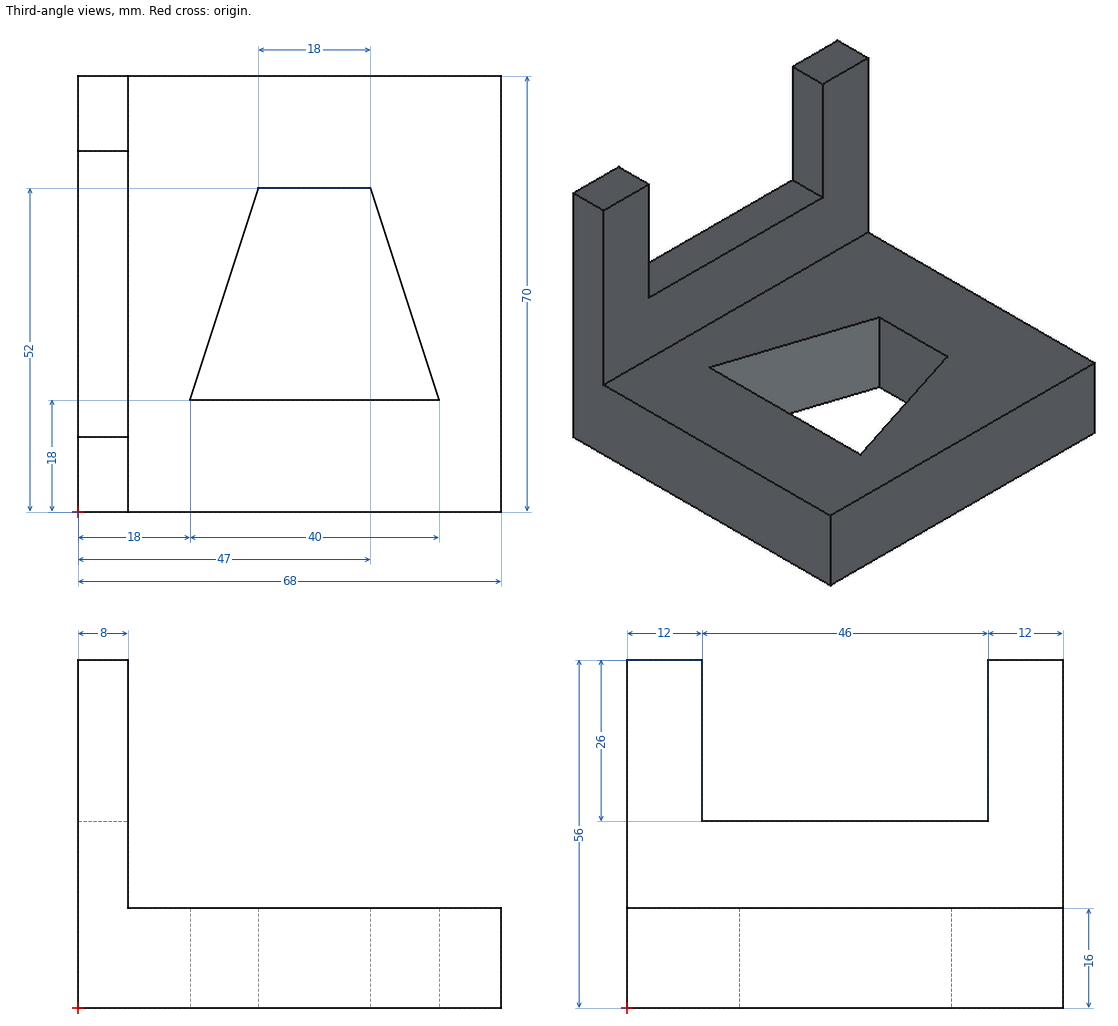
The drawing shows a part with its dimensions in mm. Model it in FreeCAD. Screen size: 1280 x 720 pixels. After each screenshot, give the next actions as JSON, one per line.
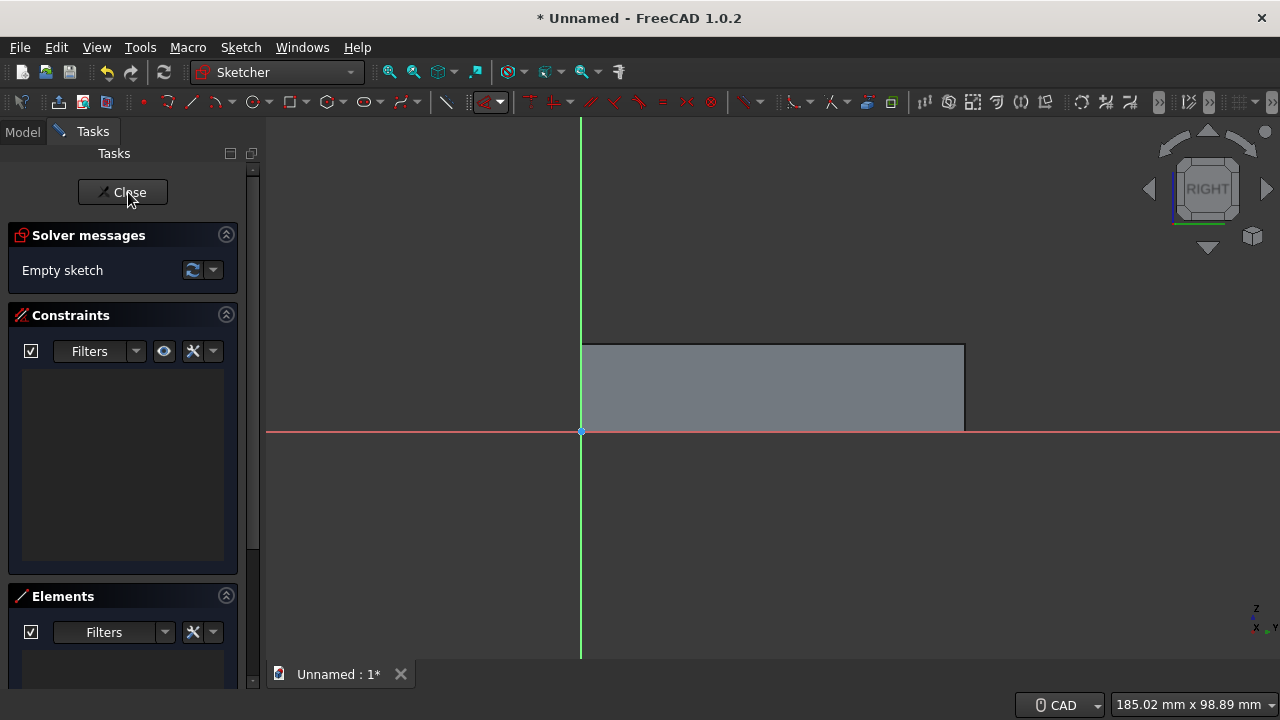
{"action": "scroll", "coordinate": [395, 631], "scroll_direction": "down", "scroll_amount": 1}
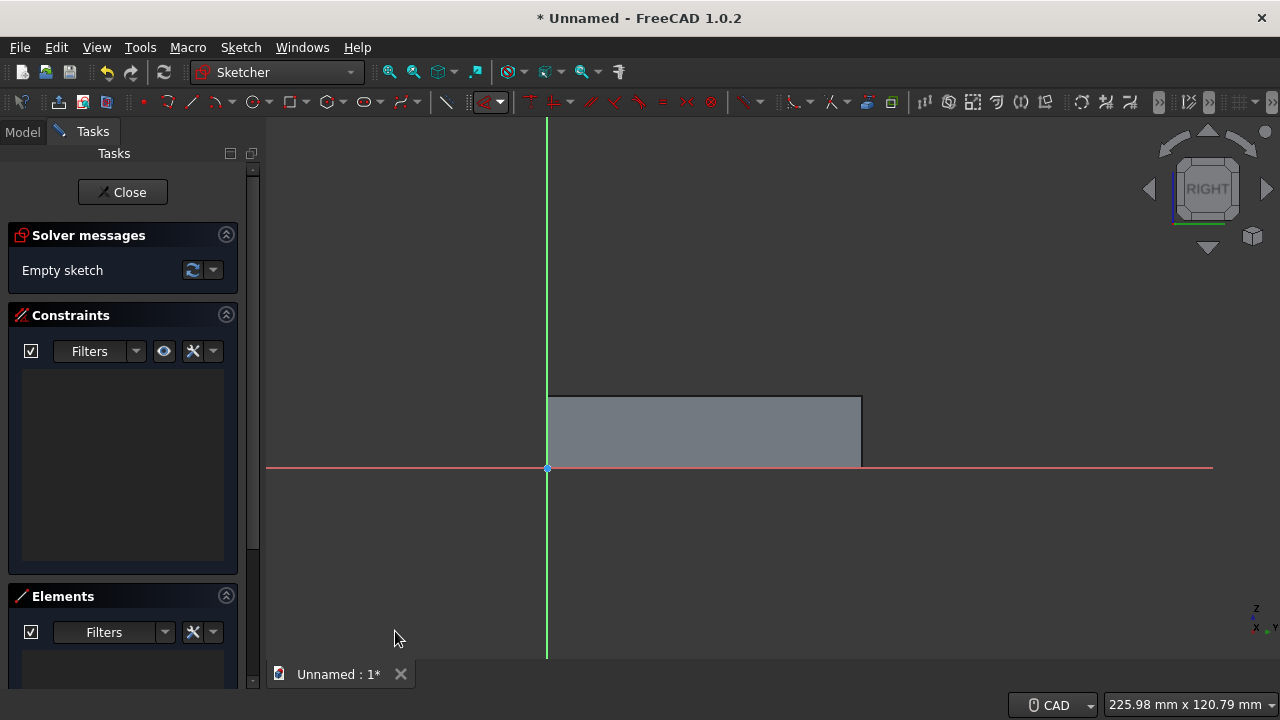
{"action": "scroll", "coordinate": [705, 250], "scroll_direction": "up", "scroll_amount": 2}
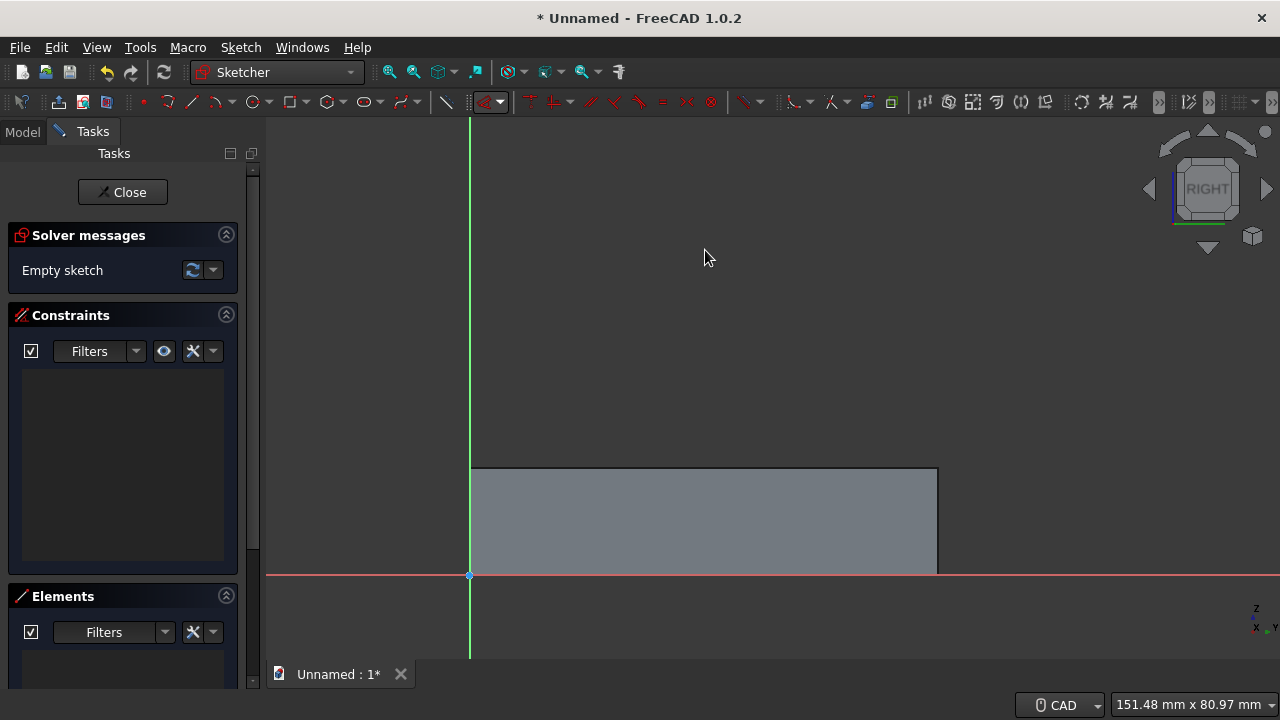
{"action": "left_click", "coordinate": [168, 102]}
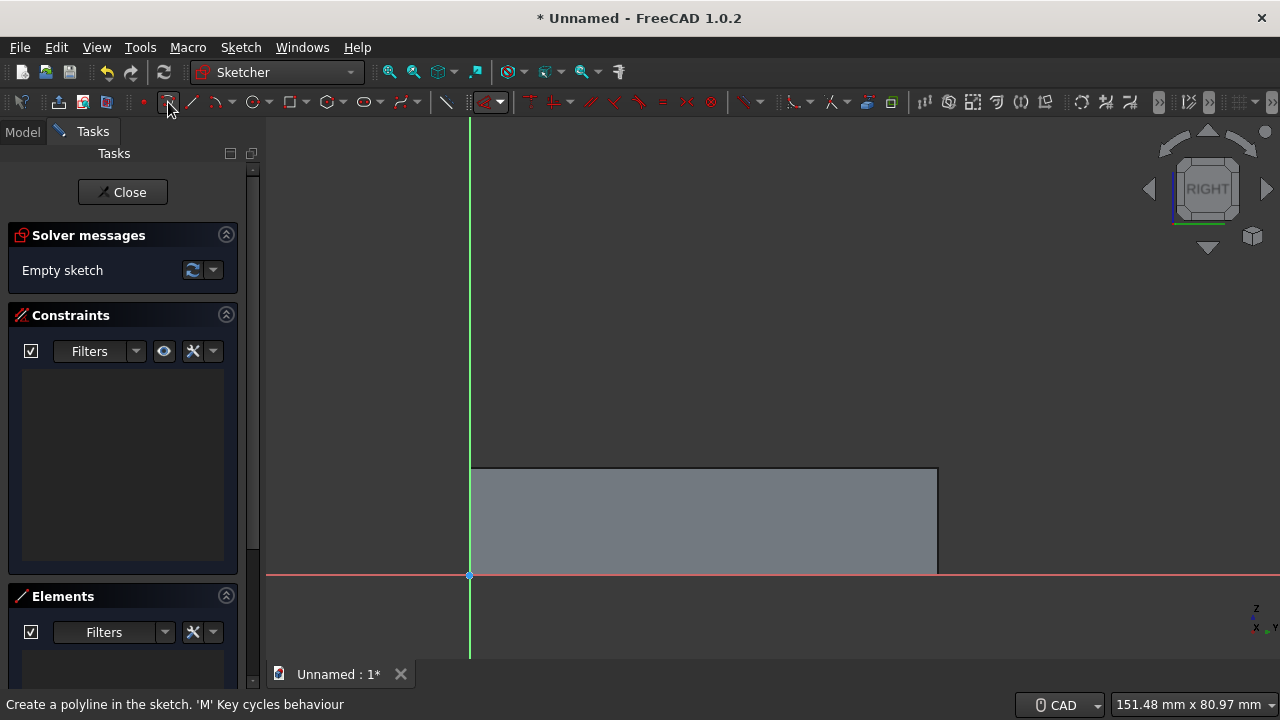
{"action": "left_click", "coordinate": [470, 575]}
{"action": "left_click", "coordinate": [479, 200]}
{"action": "left_click", "coordinate": [550, 200]}
{"action": "left_click", "coordinate": [550, 374]}
{"action": "left_click", "coordinate": [858, 374]}
{"action": "left_click", "coordinate": [858, 200]}
{"action": "left_click", "coordinate": [938, 200]}
{"action": "left_click", "coordinate": [938, 566]}
{"action": "left_click", "coordinate": [470, 575]}
{"action": "key", "text": "Escape"}
{"action": "key", "text": "Escape"}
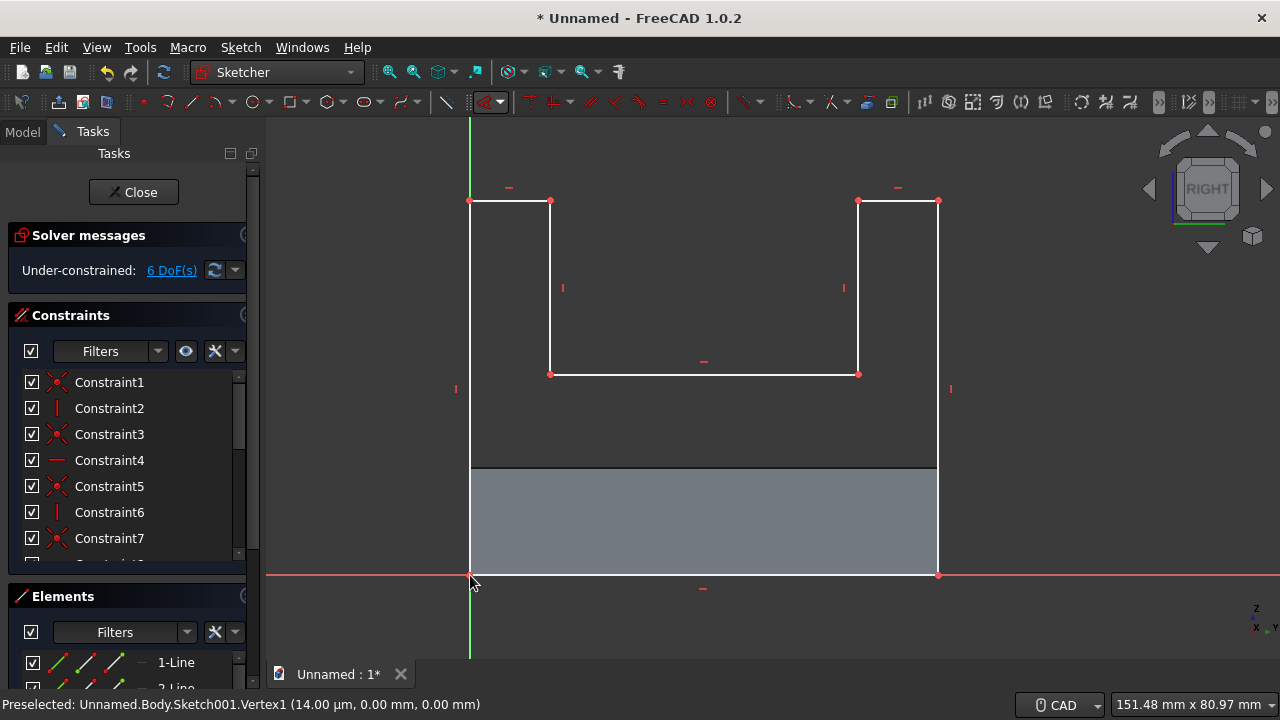
{"action": "left_click", "coordinate": [470, 463]}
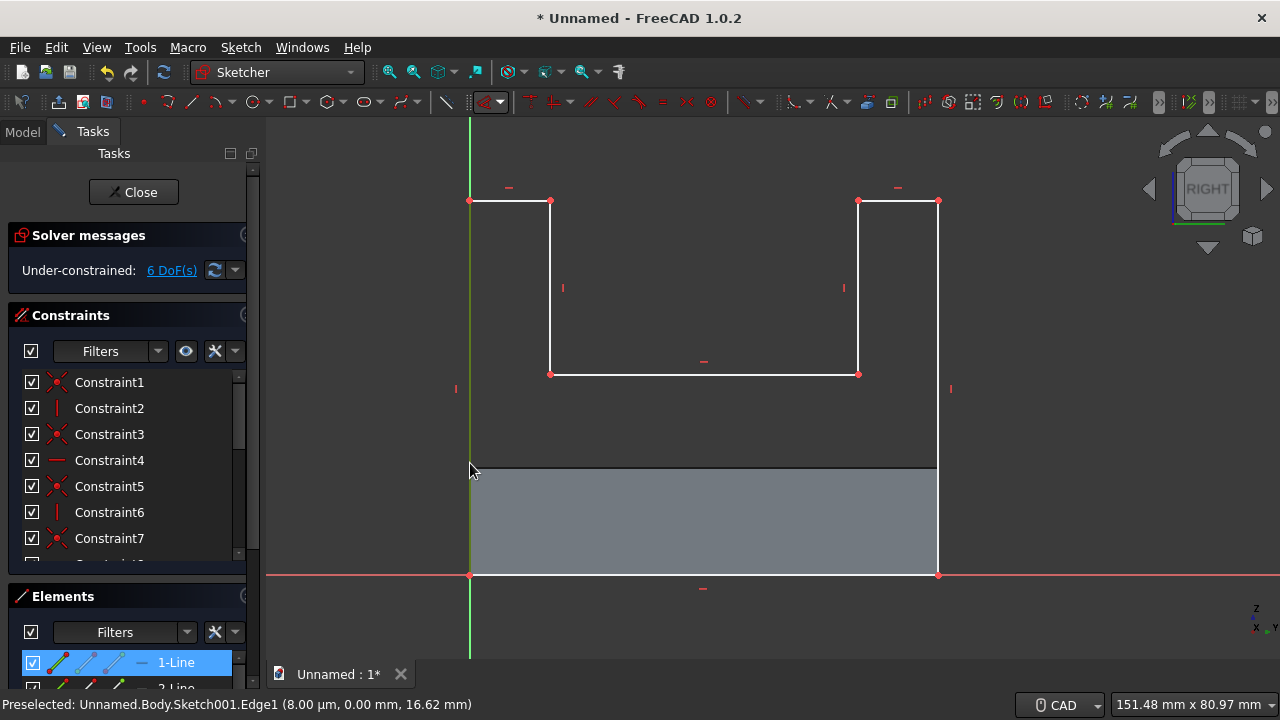
{"action": "key", "text": "i"}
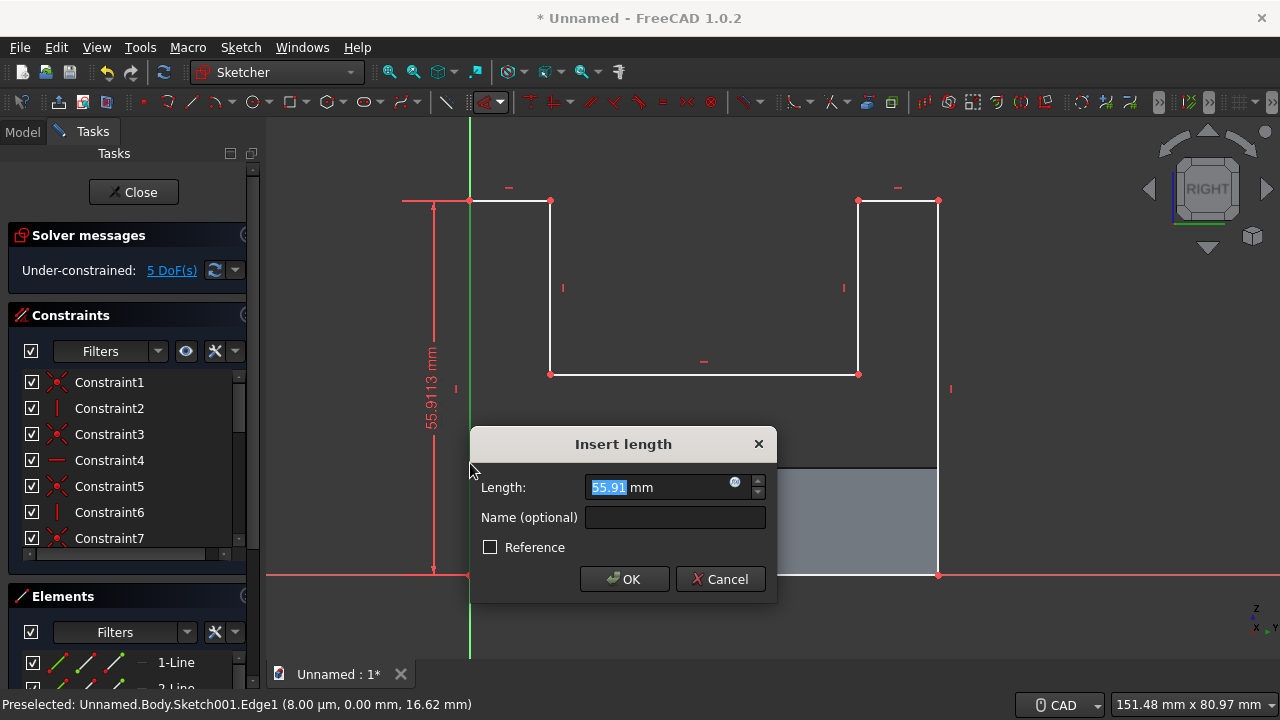
{"action": "type", "text": "56"}
{"action": "key", "text": "Return"}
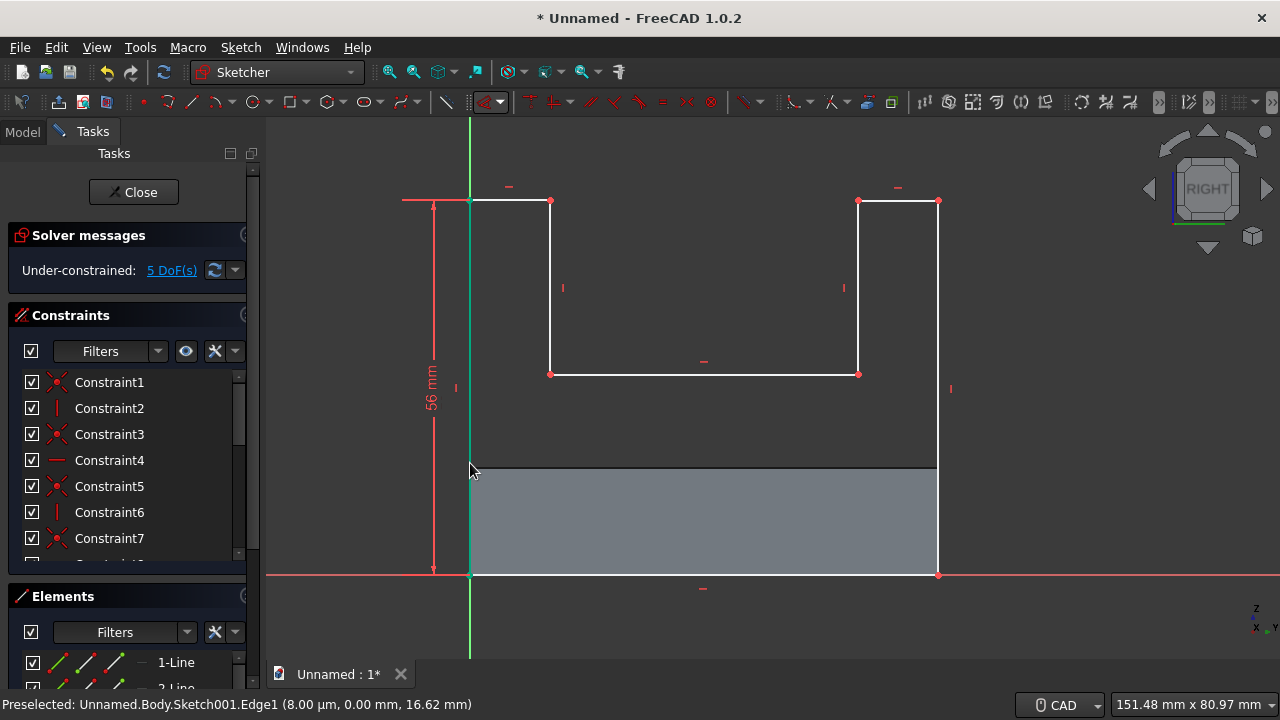
{"action": "left_click", "coordinate": [494, 200]}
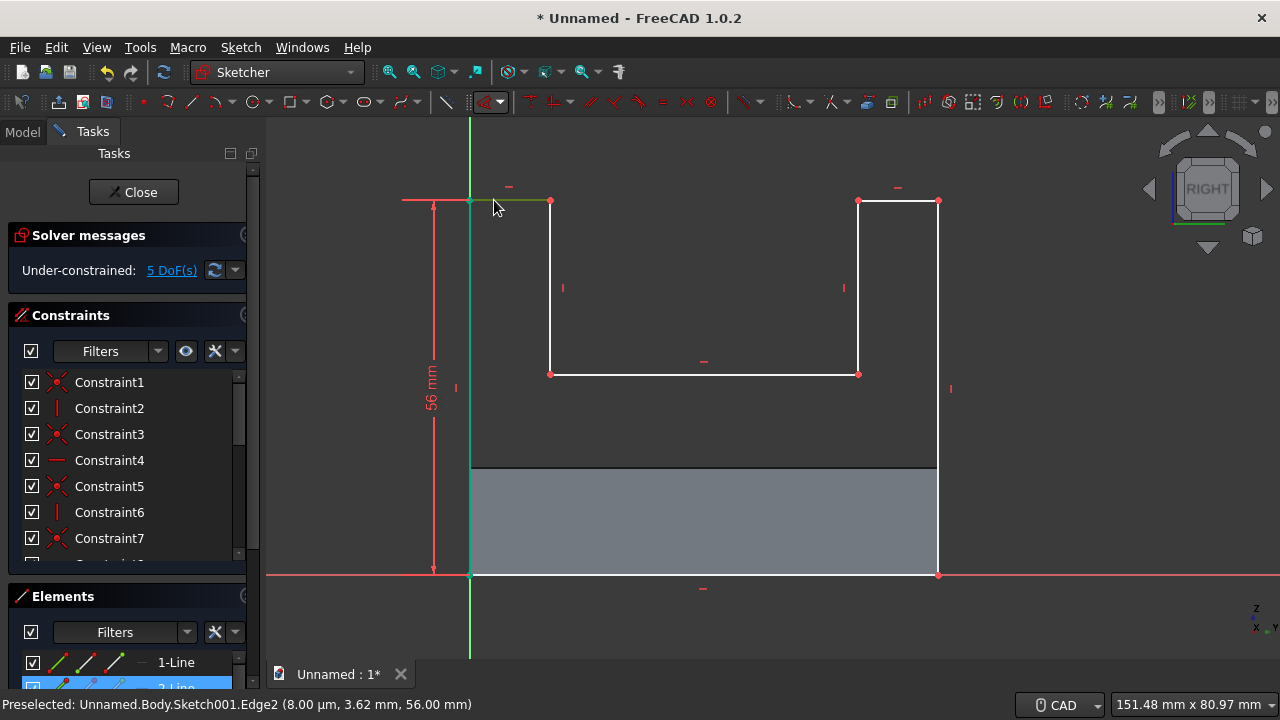
{"action": "key", "text": "l"}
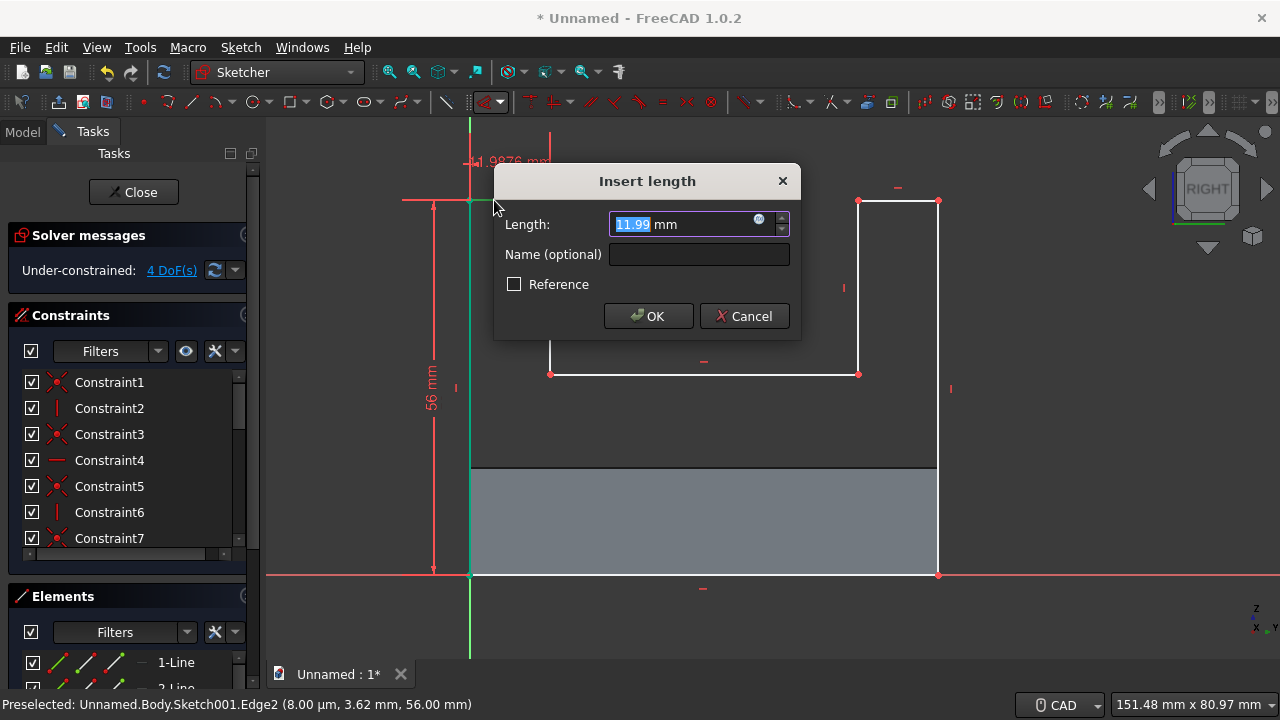
{"action": "type", "text": "12"}
{"action": "key", "text": "Return"}